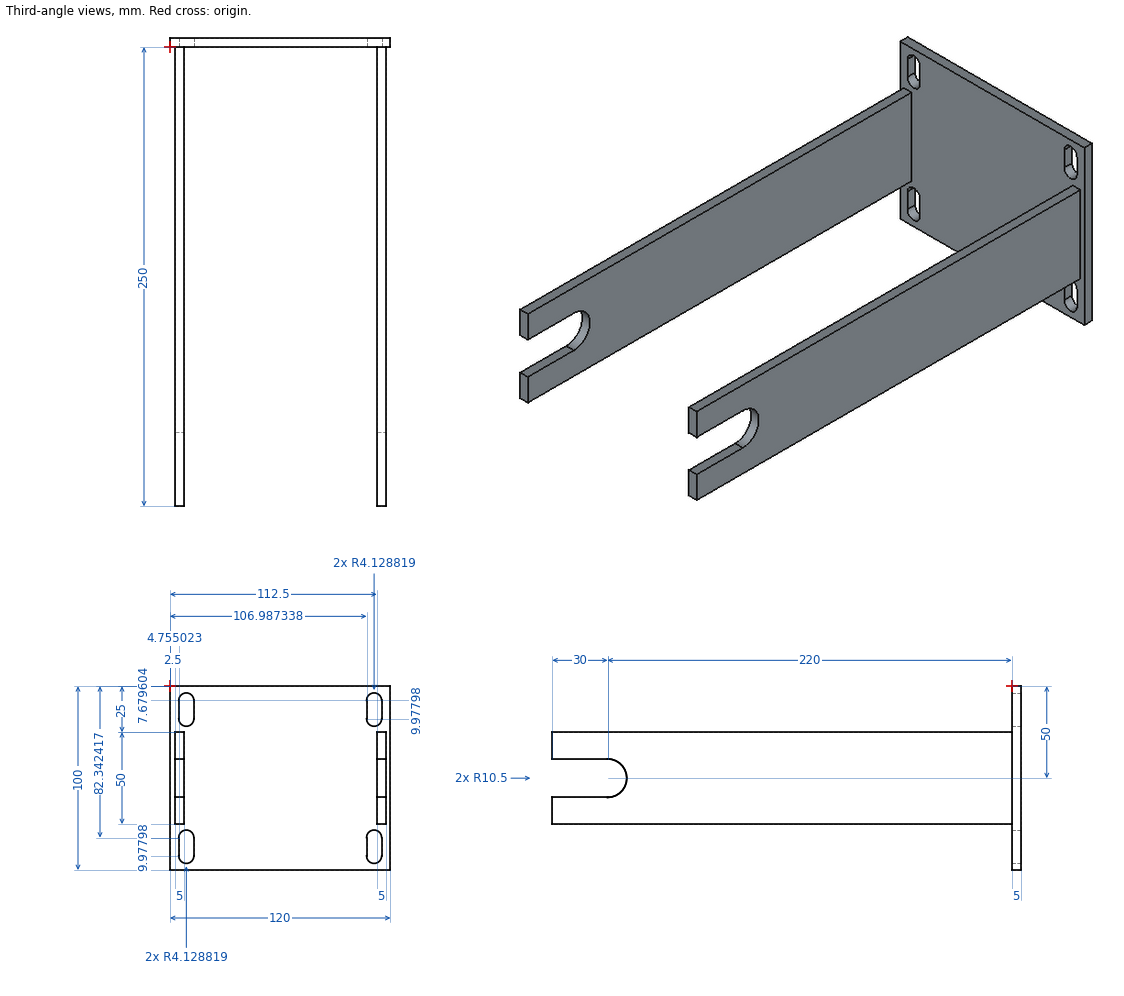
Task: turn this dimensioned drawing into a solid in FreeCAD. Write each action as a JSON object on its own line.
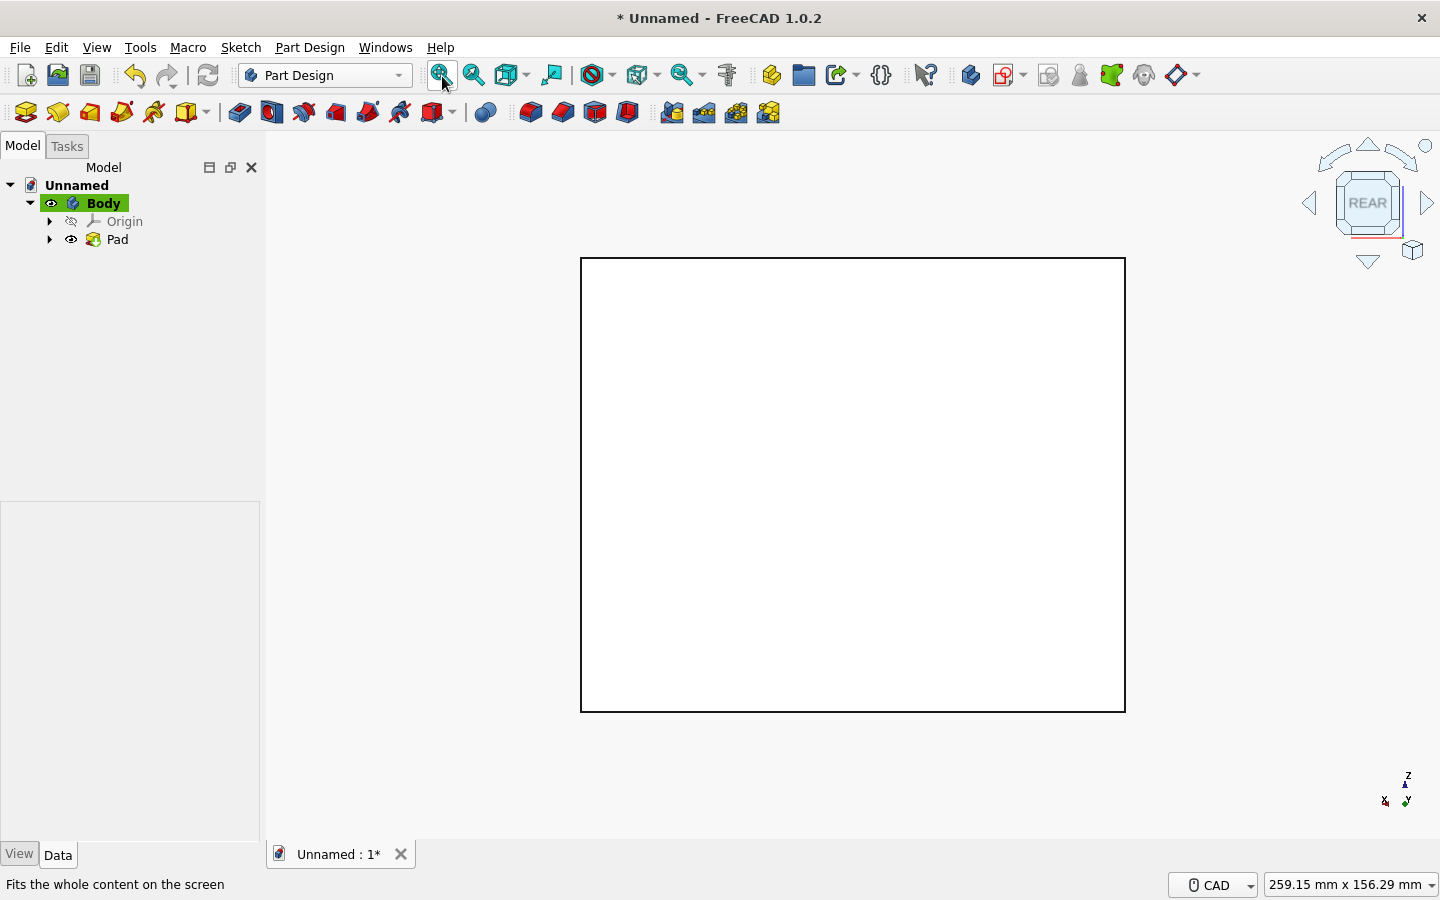
{"action": "left_click", "coordinate": [853, 484]}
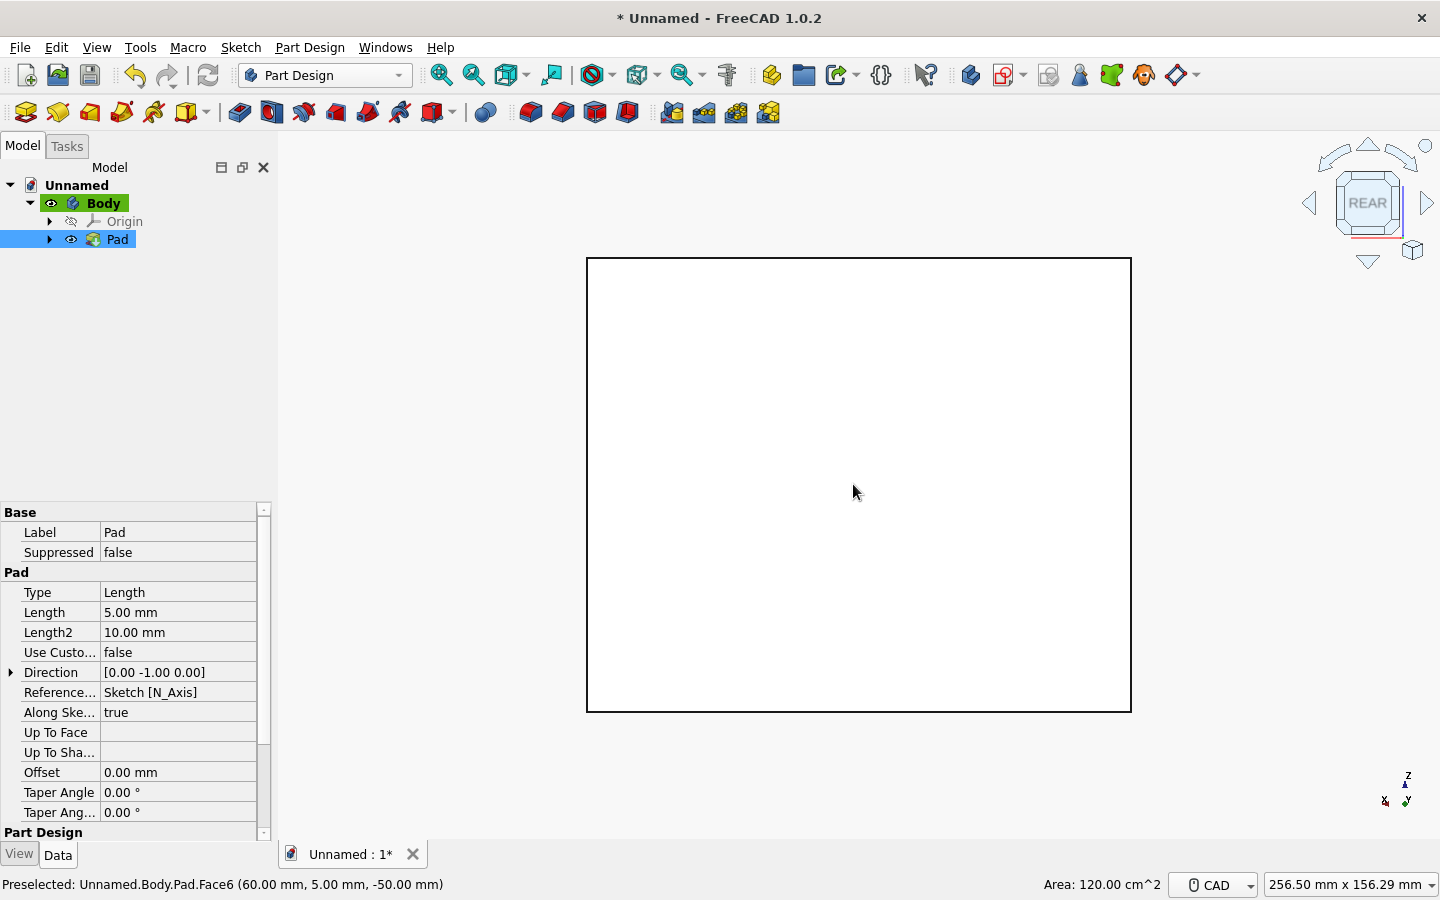
{"action": "left_click", "coordinate": [1004, 76]}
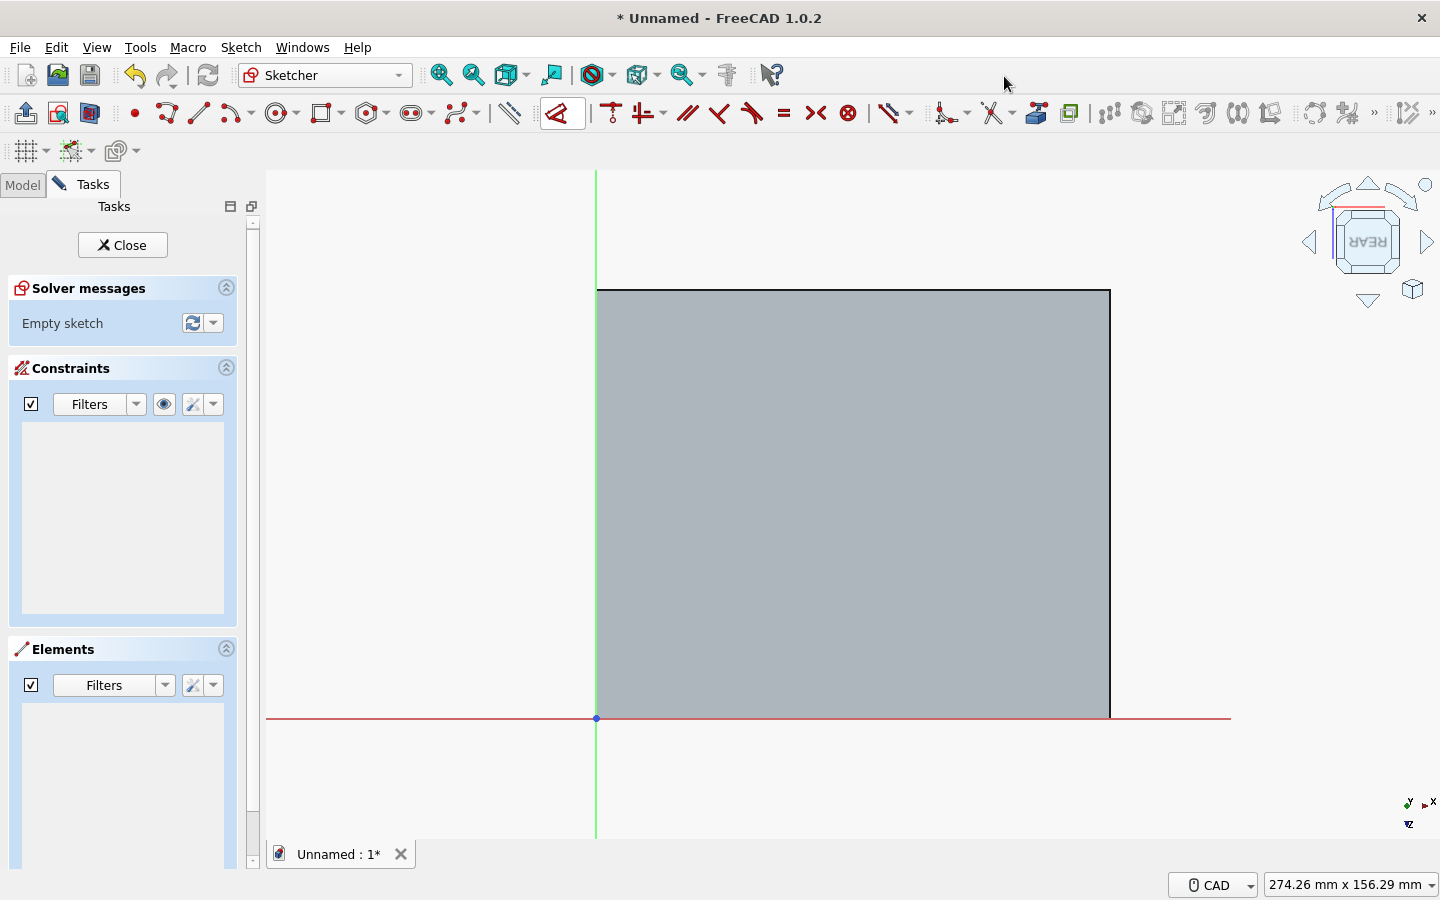
{"action": "scroll", "coordinate": [604, 313], "scroll_direction": "up", "scroll_amount": 9}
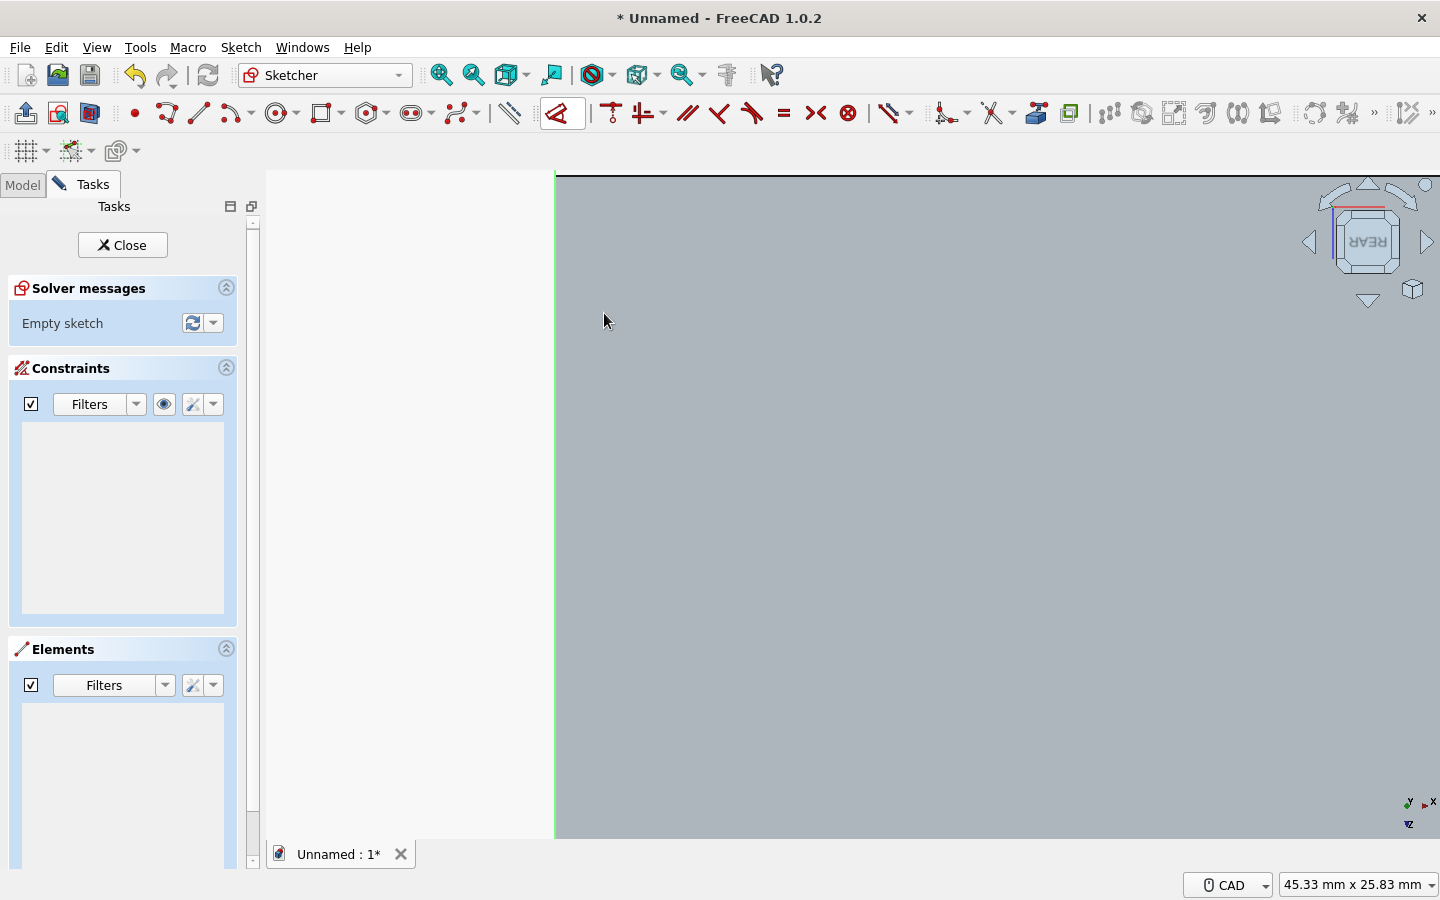
{"action": "left_click", "coordinate": [412, 114]}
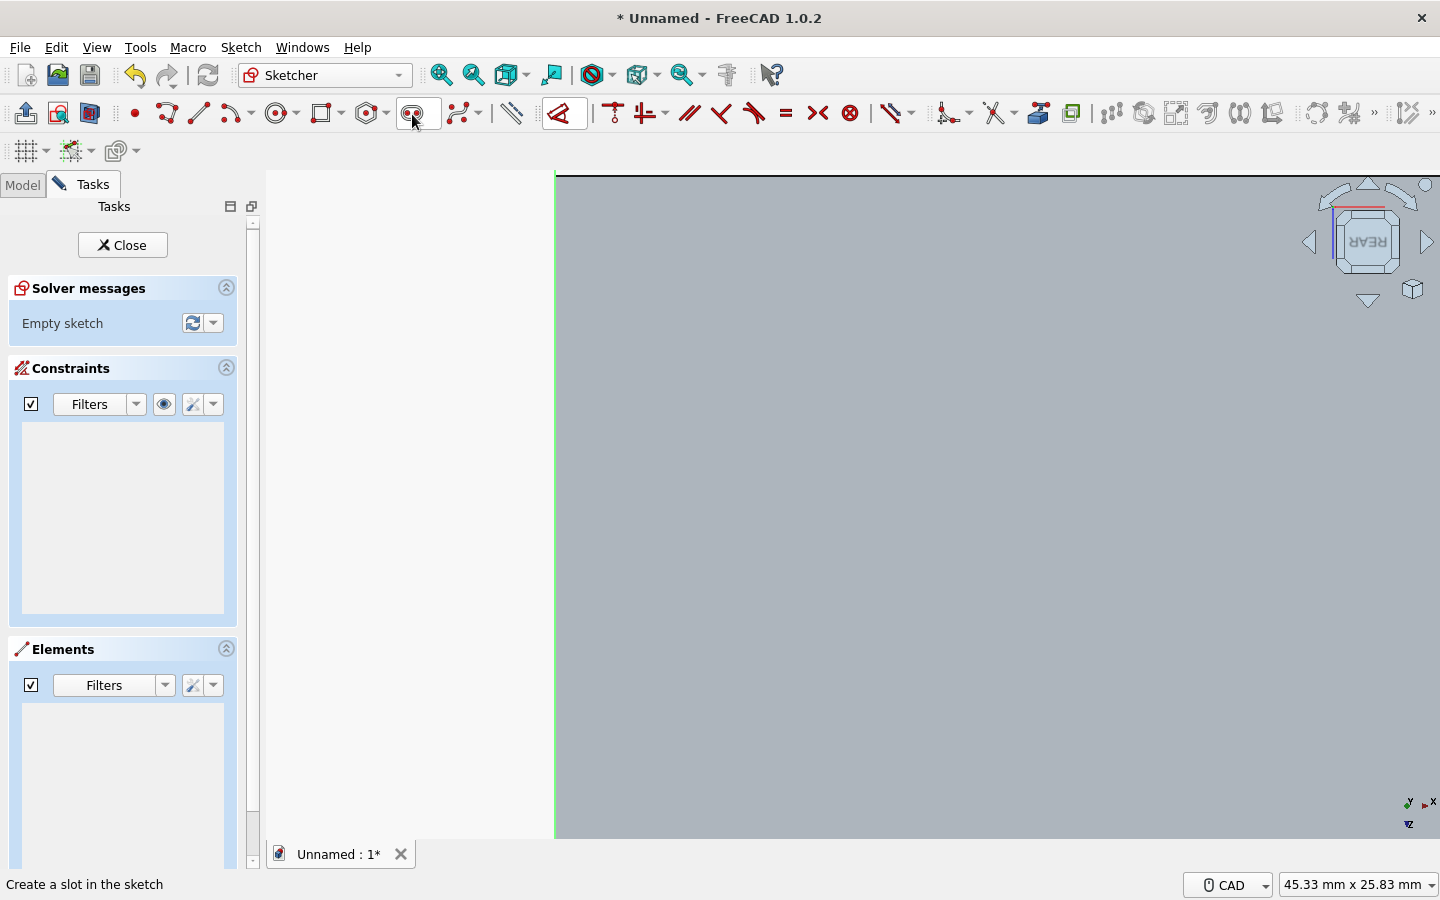
{"action": "left_click", "coordinate": [785, 633]}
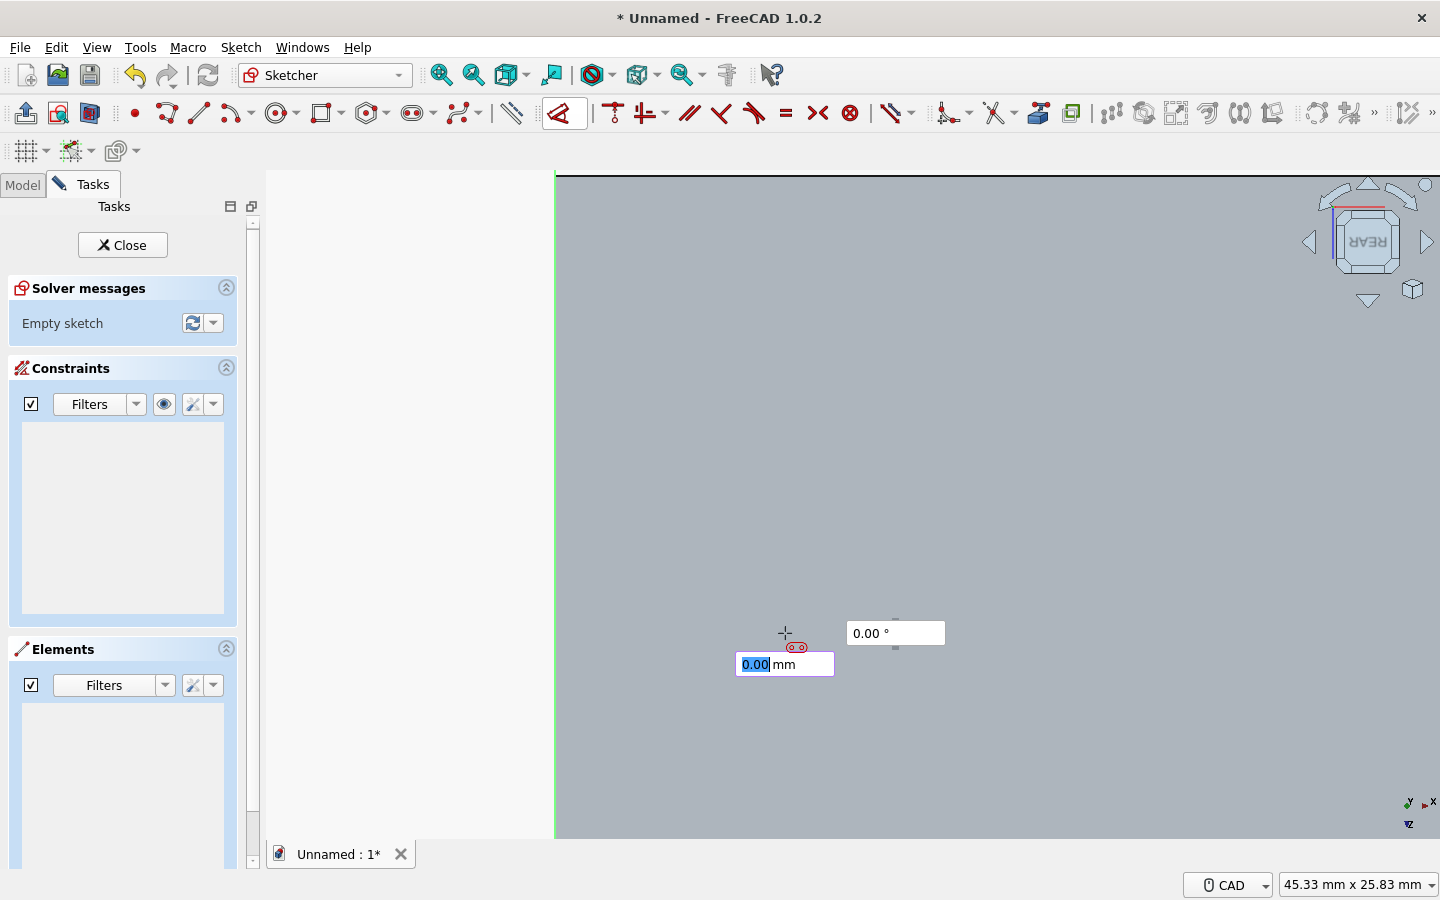
{"action": "left_click", "coordinate": [785, 374]}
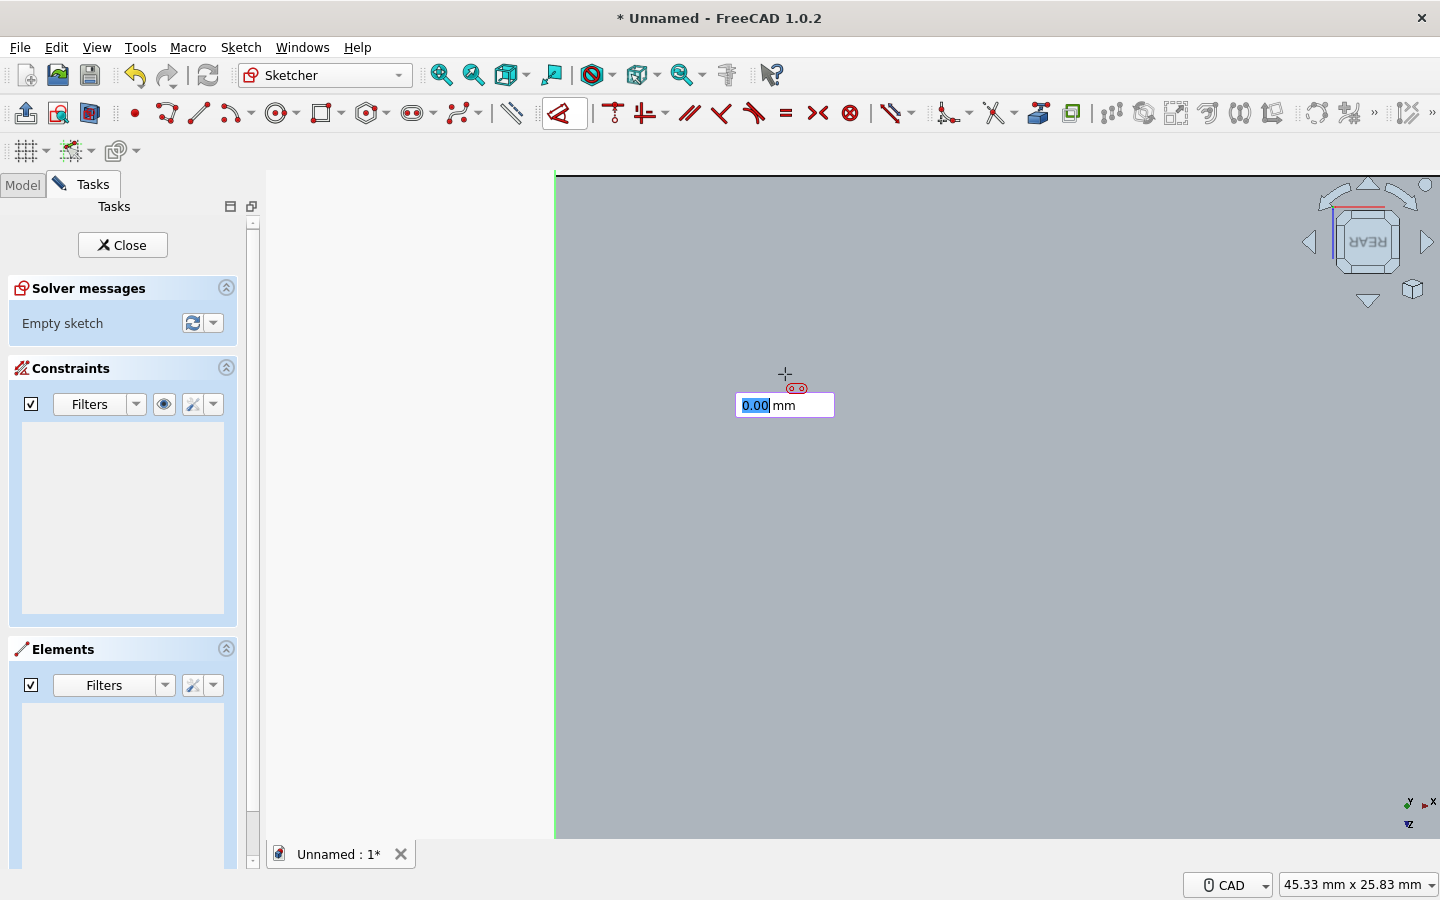
{"action": "left_click", "coordinate": [892, 504]}
{"action": "key", "text": "Escape"}